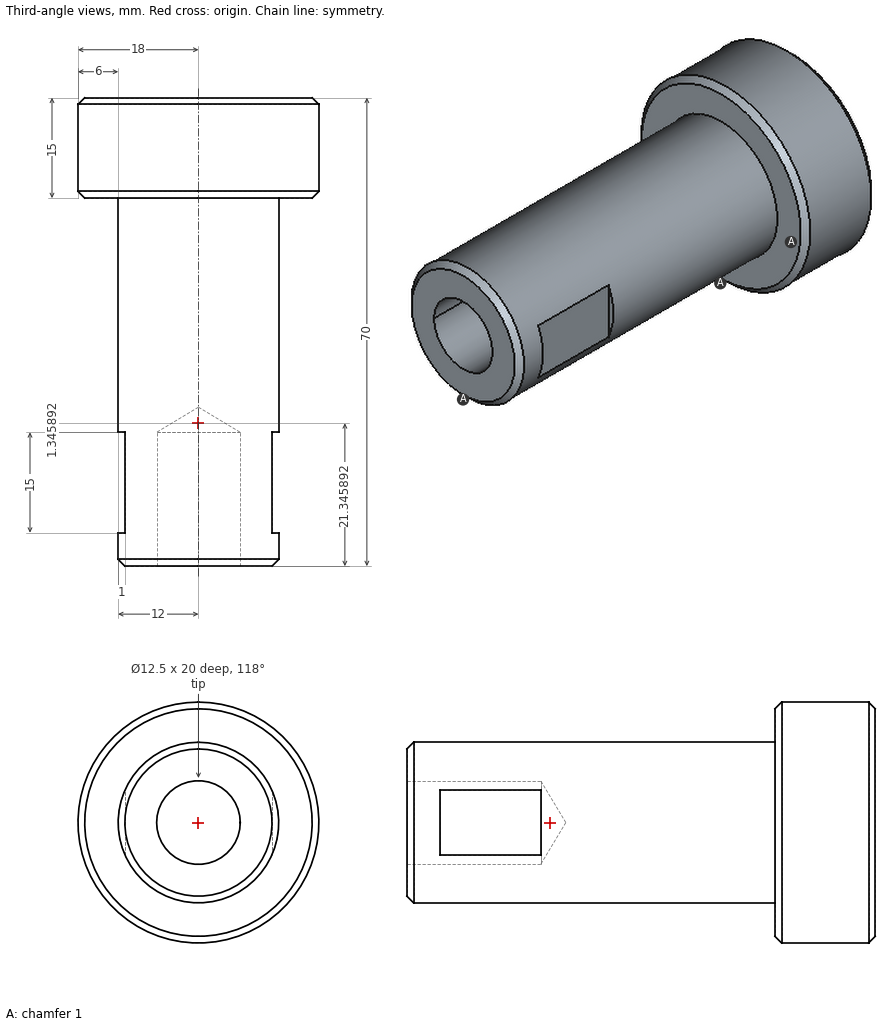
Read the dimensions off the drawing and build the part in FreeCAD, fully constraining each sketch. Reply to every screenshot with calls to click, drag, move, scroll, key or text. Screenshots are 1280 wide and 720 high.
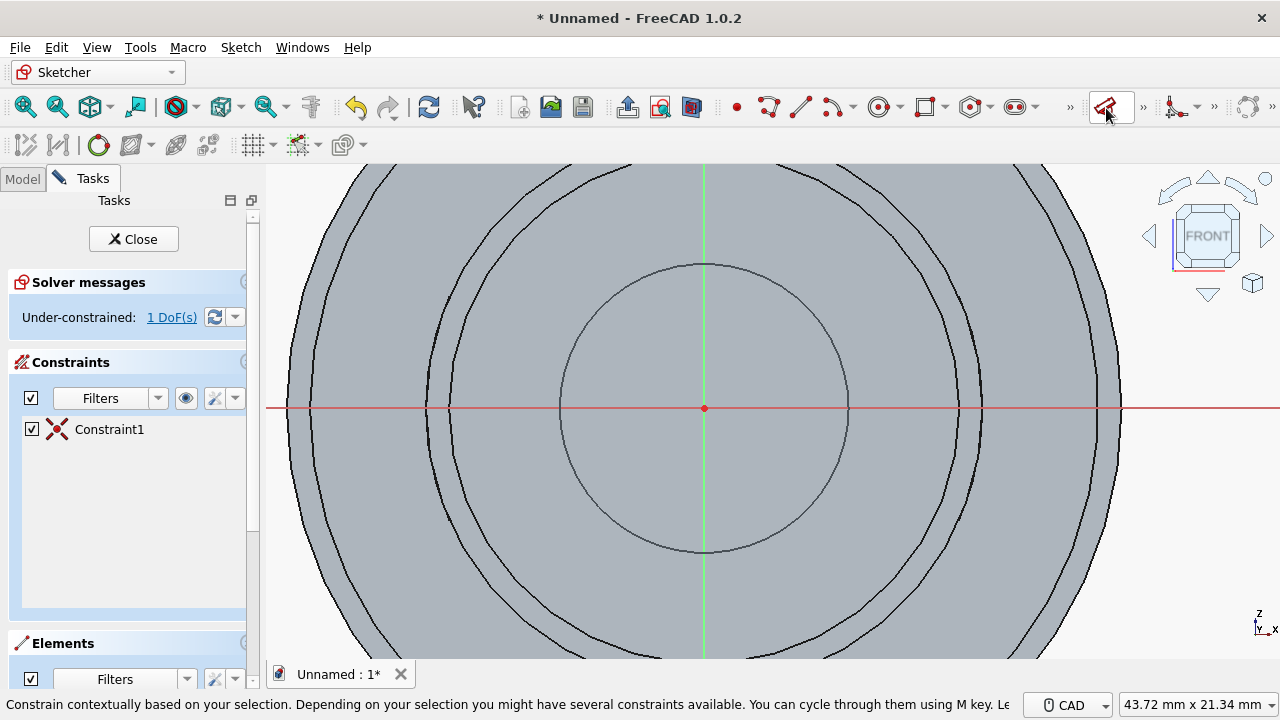
click(806, 306)
click(829, 283)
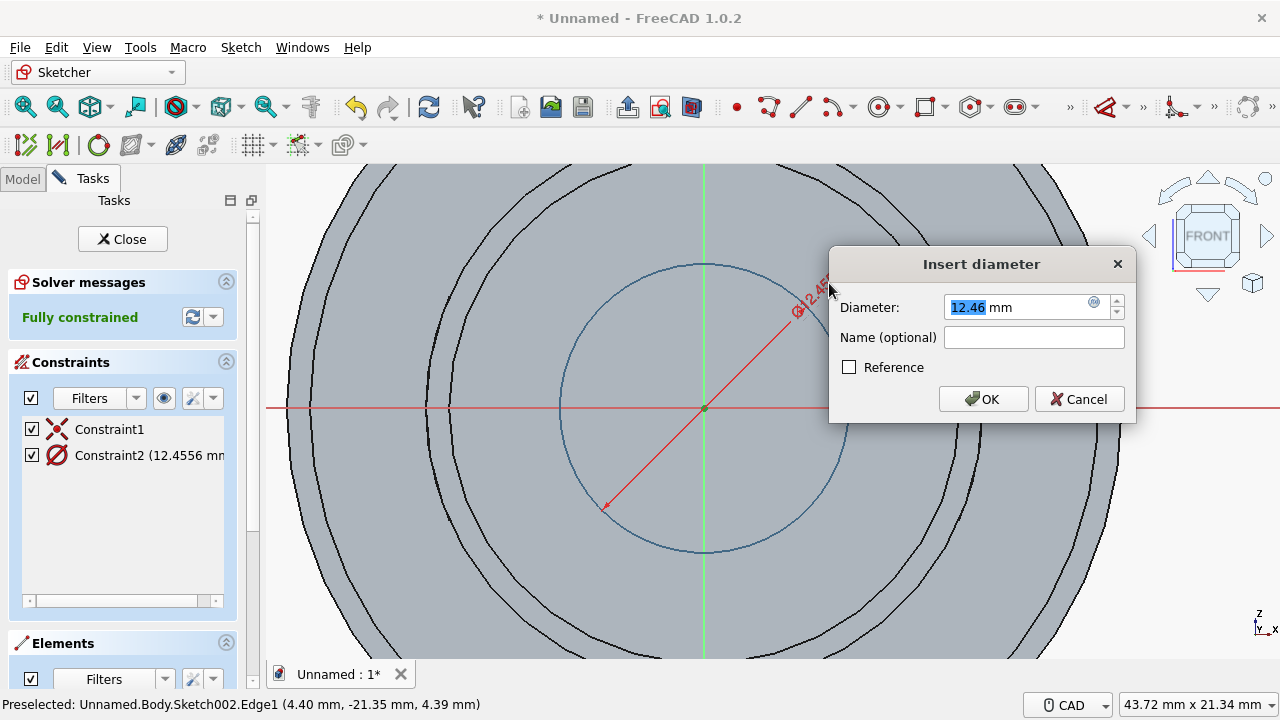
text(12.5)
key(Return)
key(Escape)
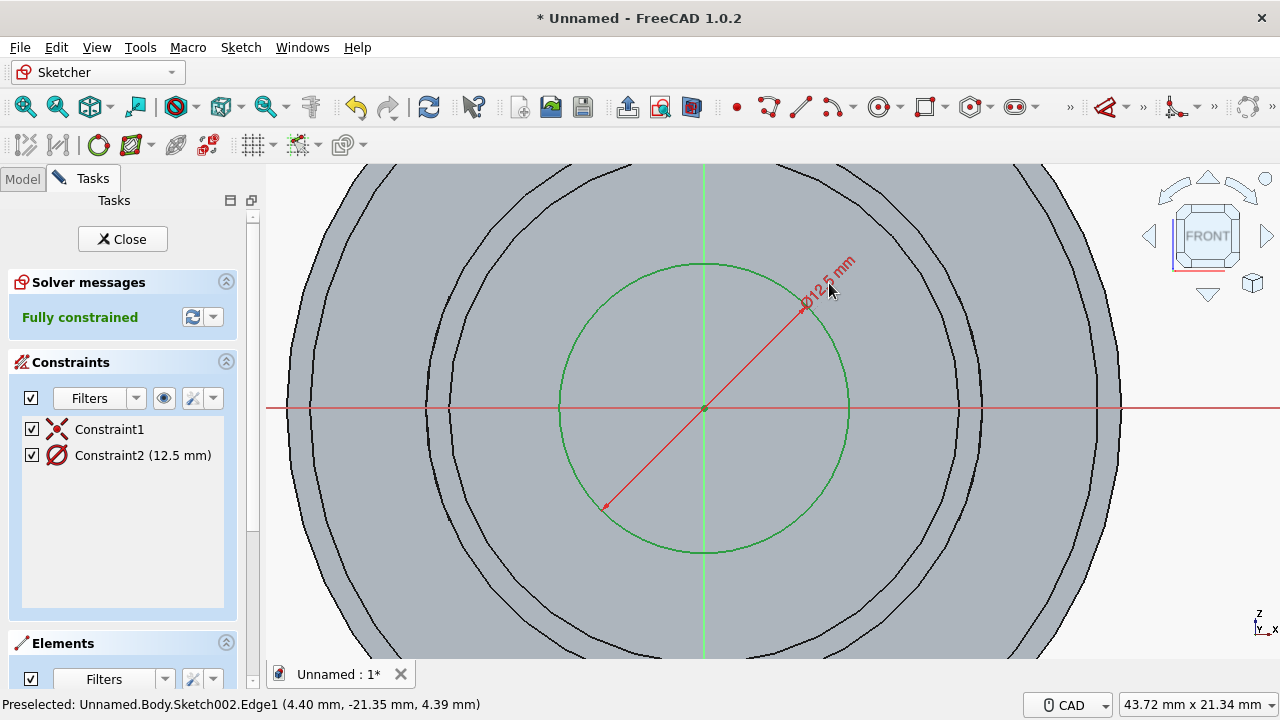
click(123, 239)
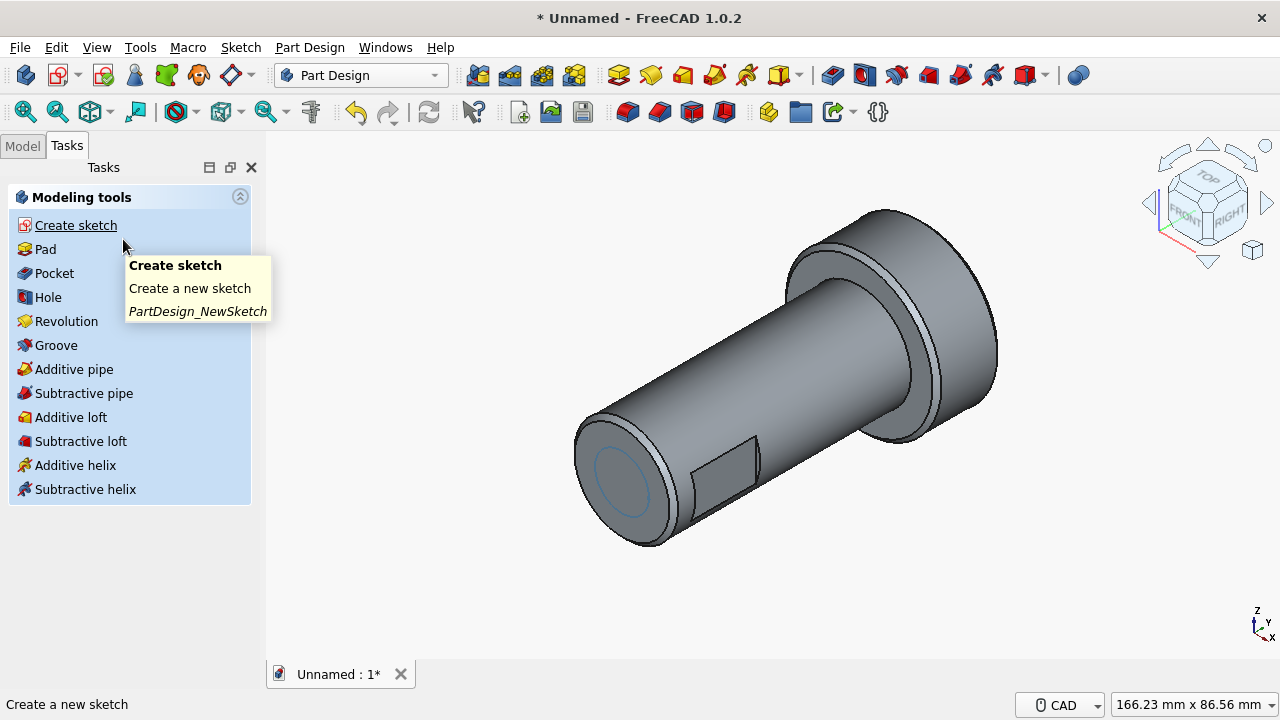
click(866, 76)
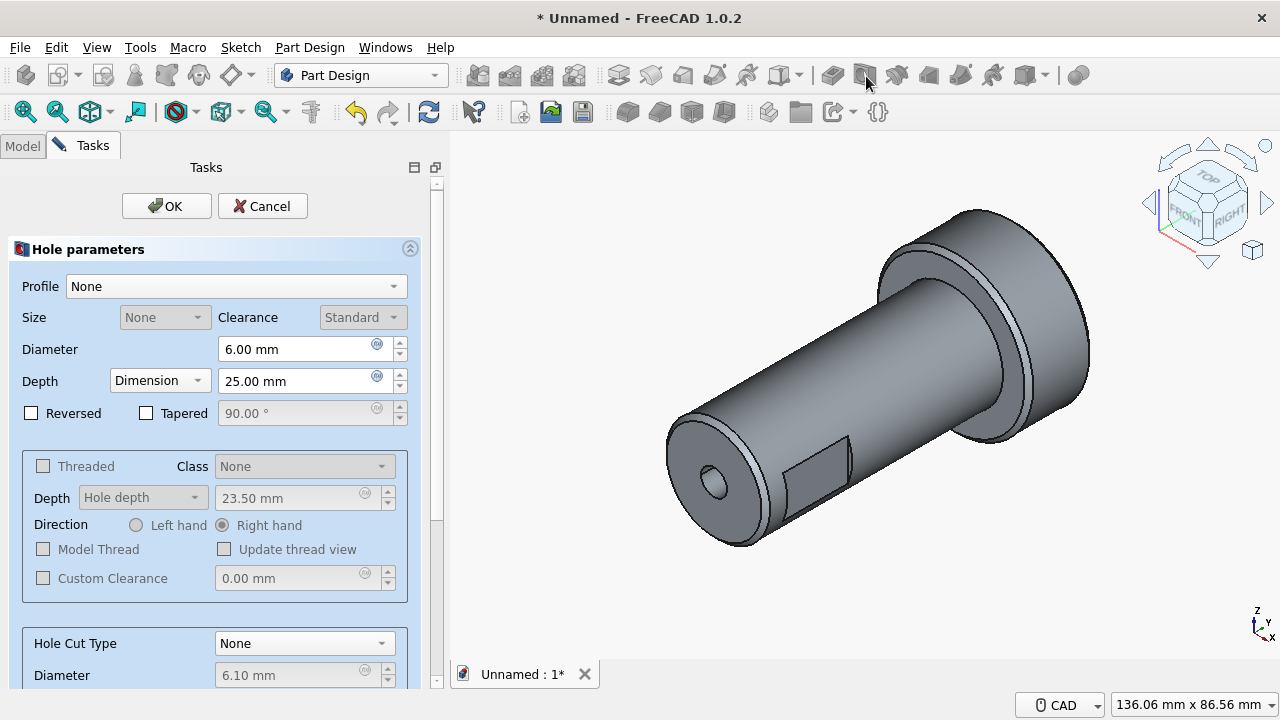
triple_click(305, 349)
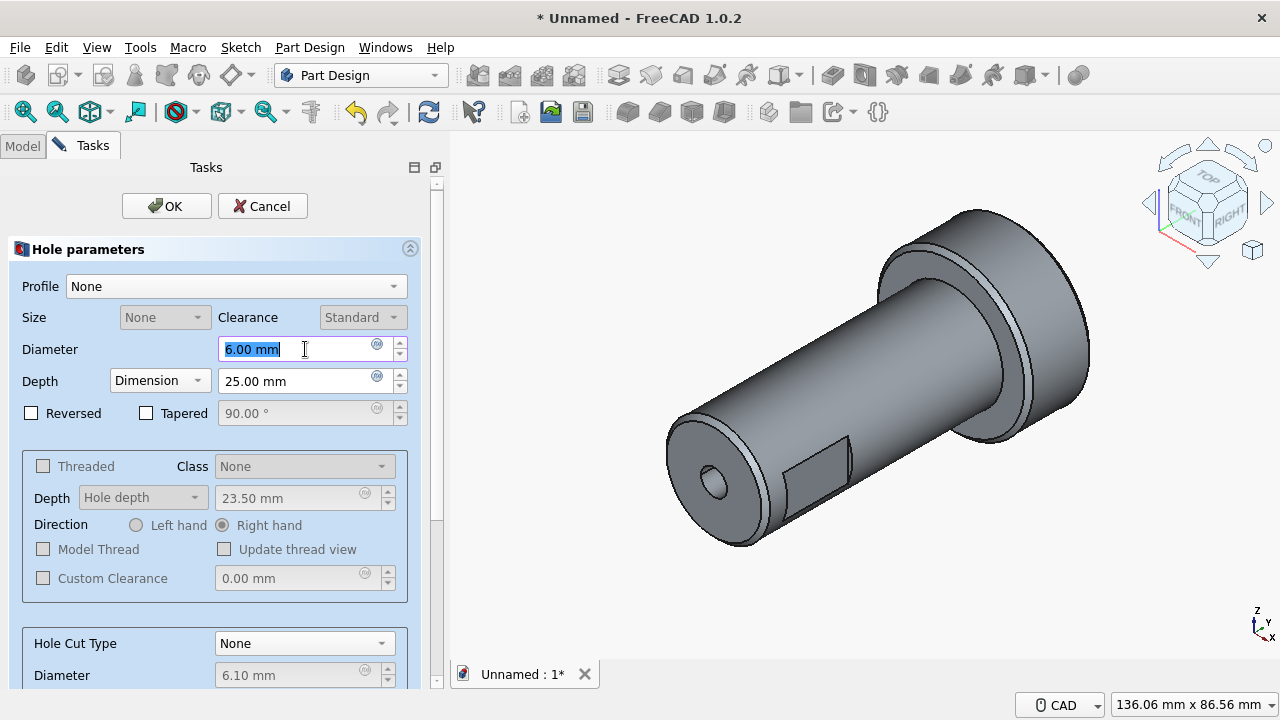
text(12.5)
key(Tab)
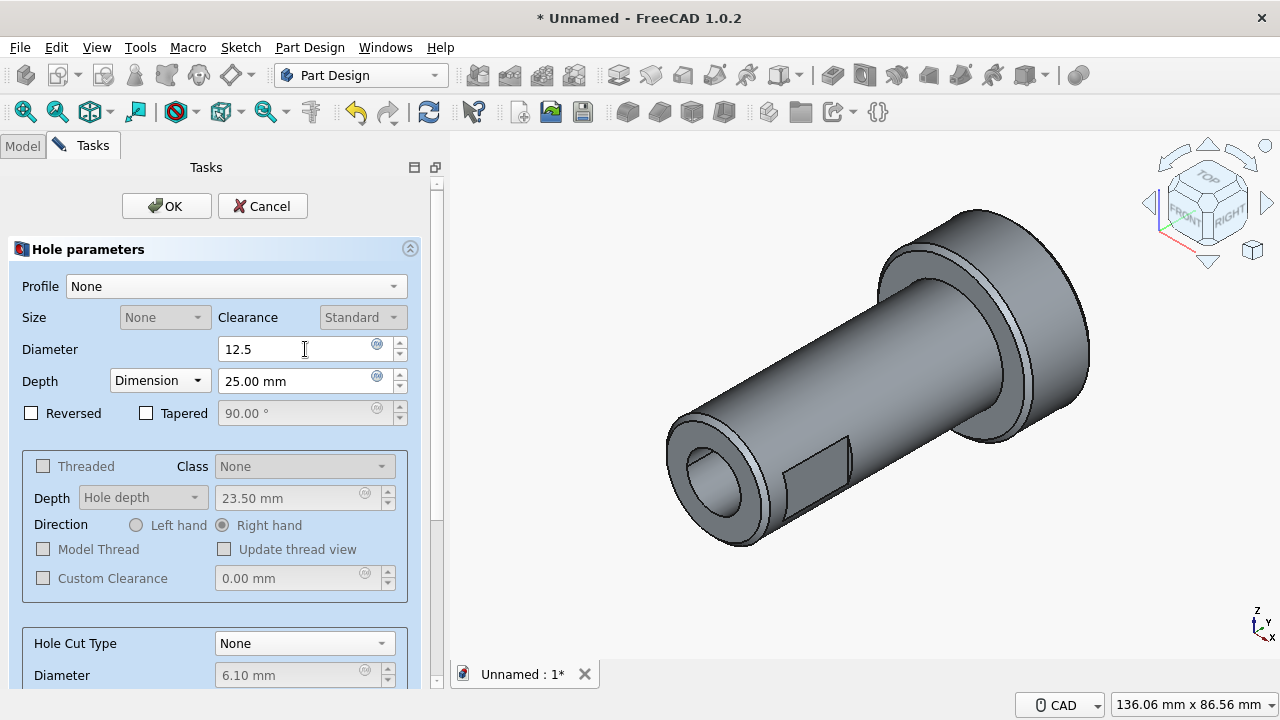
triple_click(305, 381)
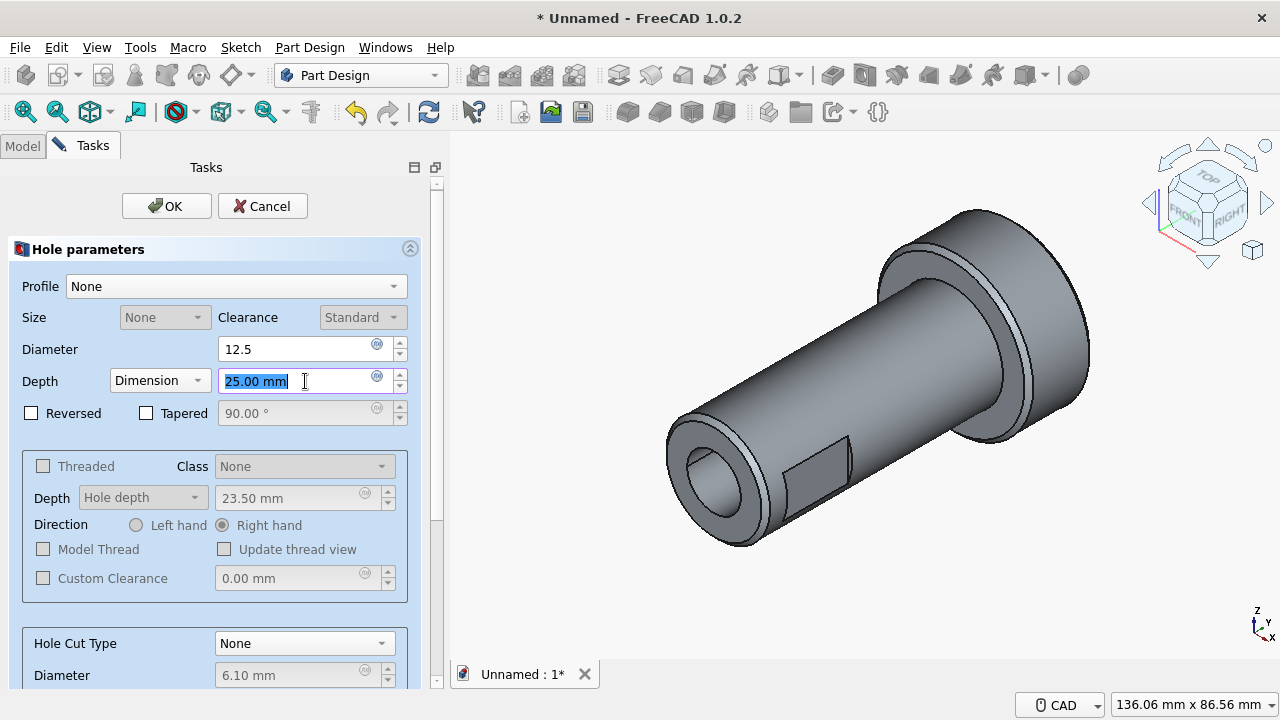
text(20)
key(Tab)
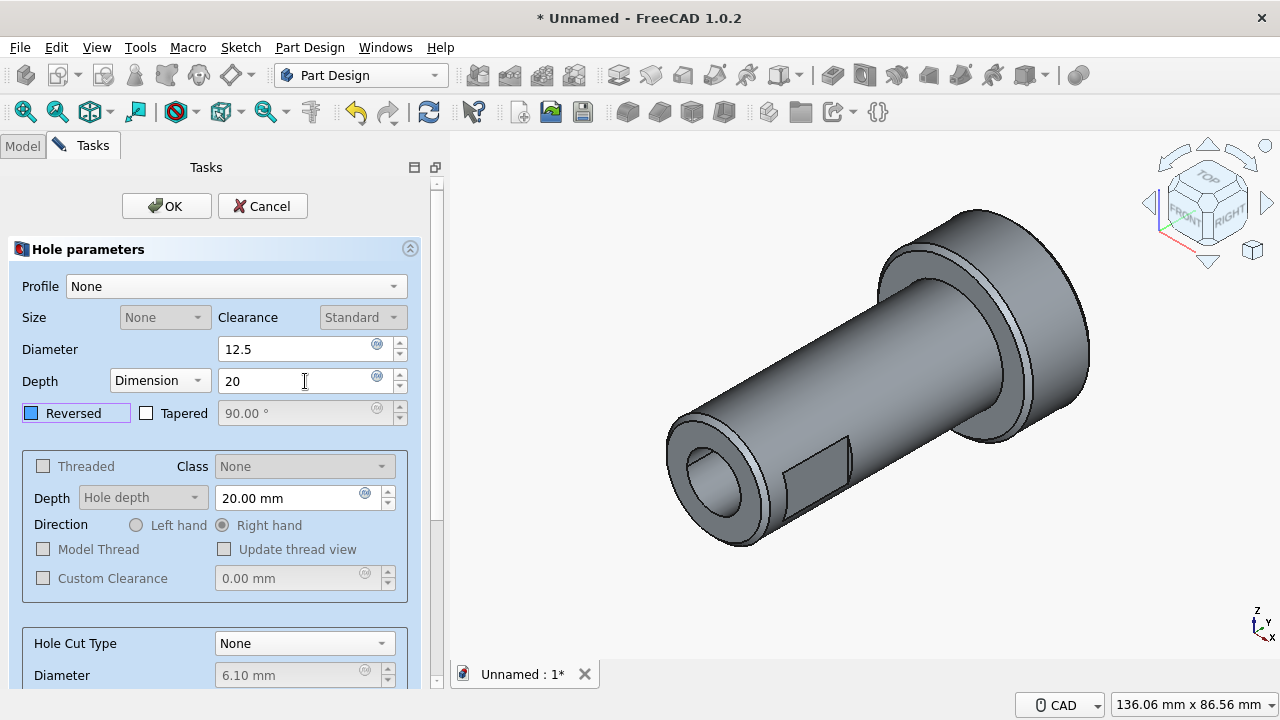
click(167, 206)